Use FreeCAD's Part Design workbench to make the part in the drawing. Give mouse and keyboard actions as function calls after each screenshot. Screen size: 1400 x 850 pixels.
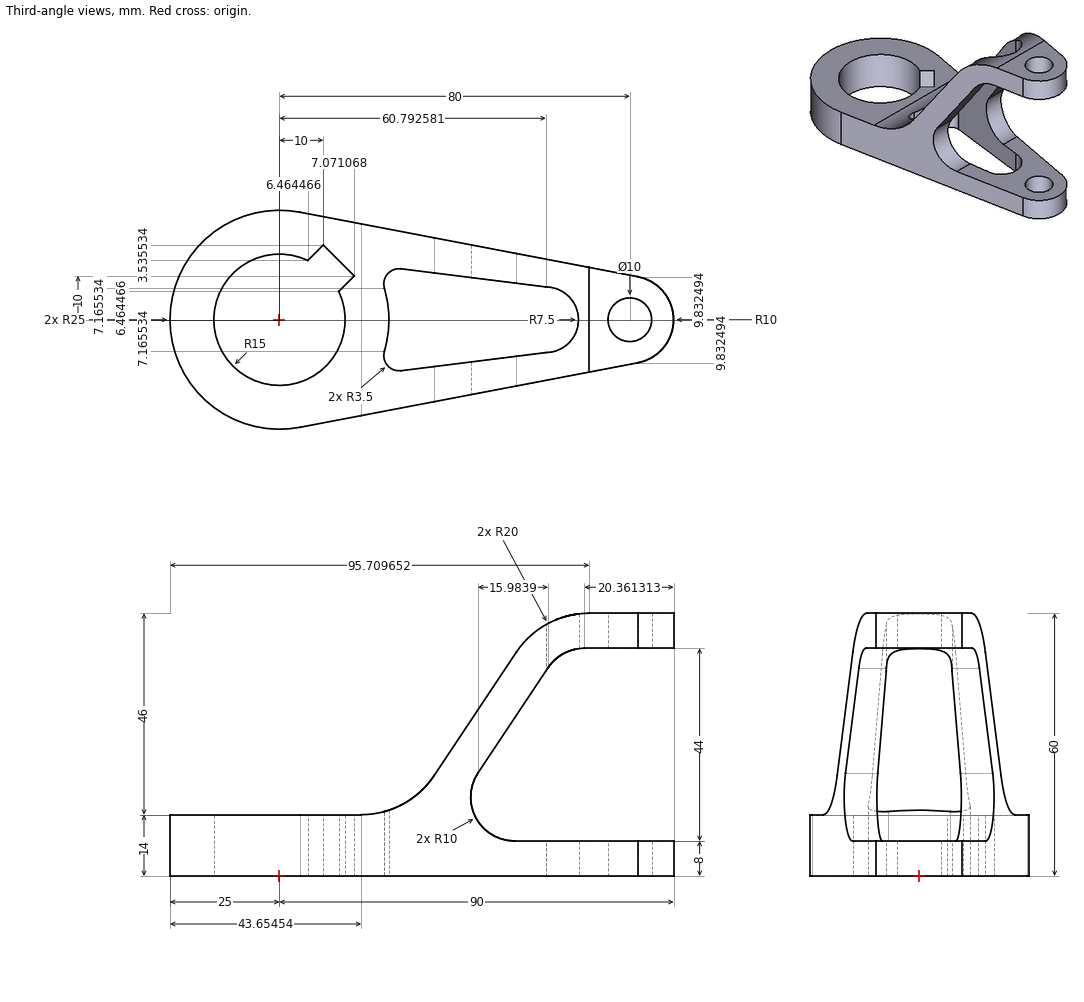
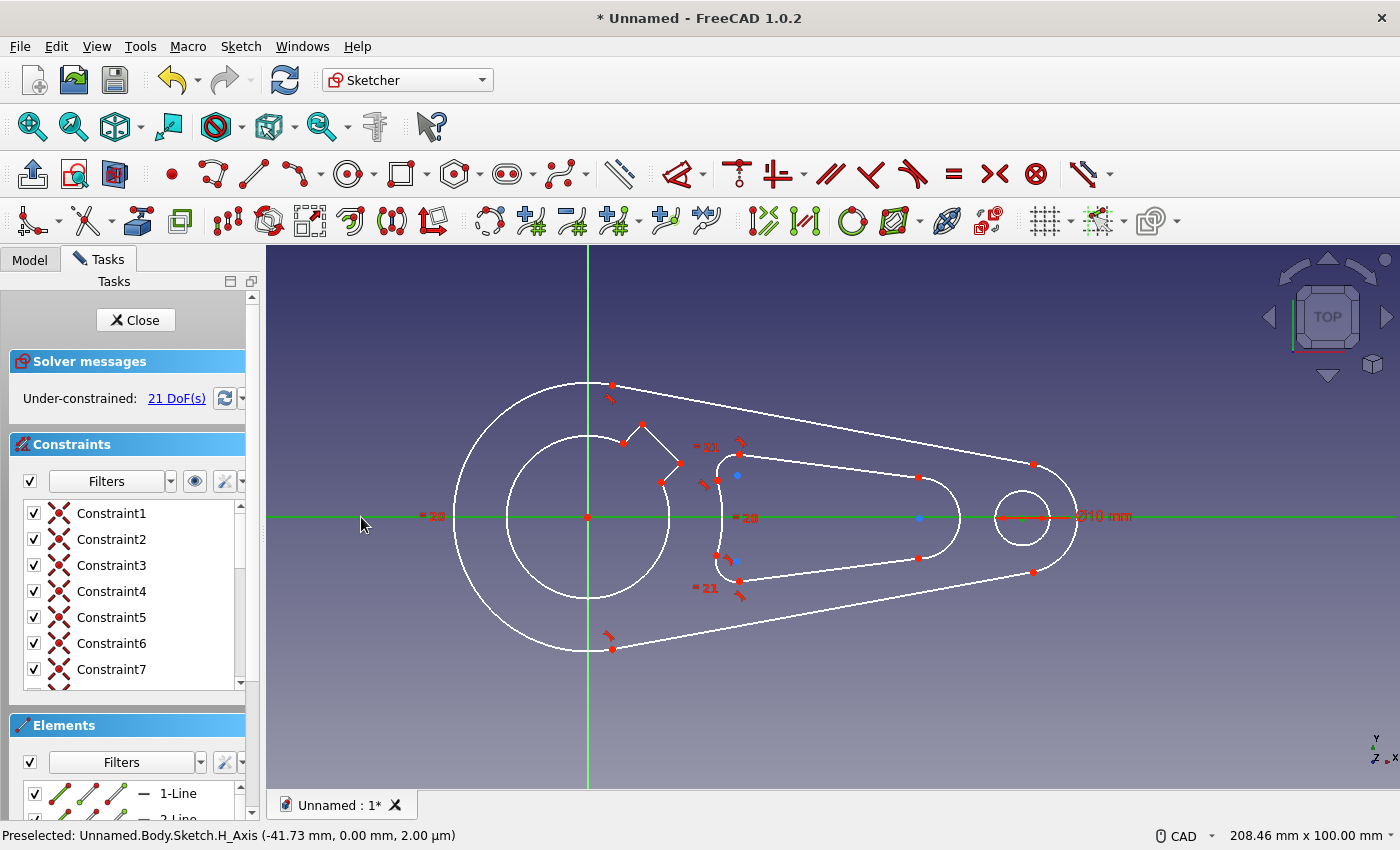
click(737, 174)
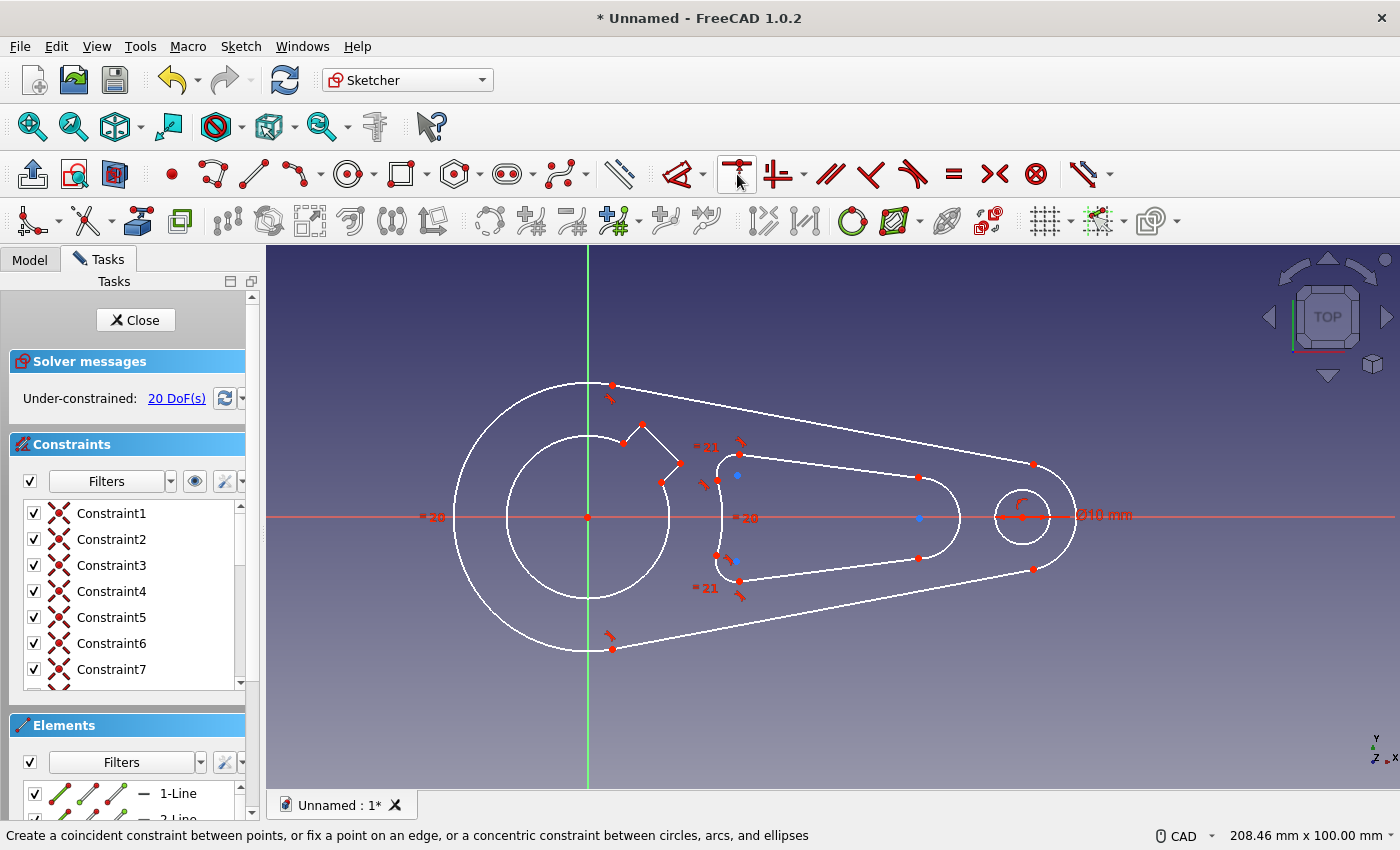
click(920, 518)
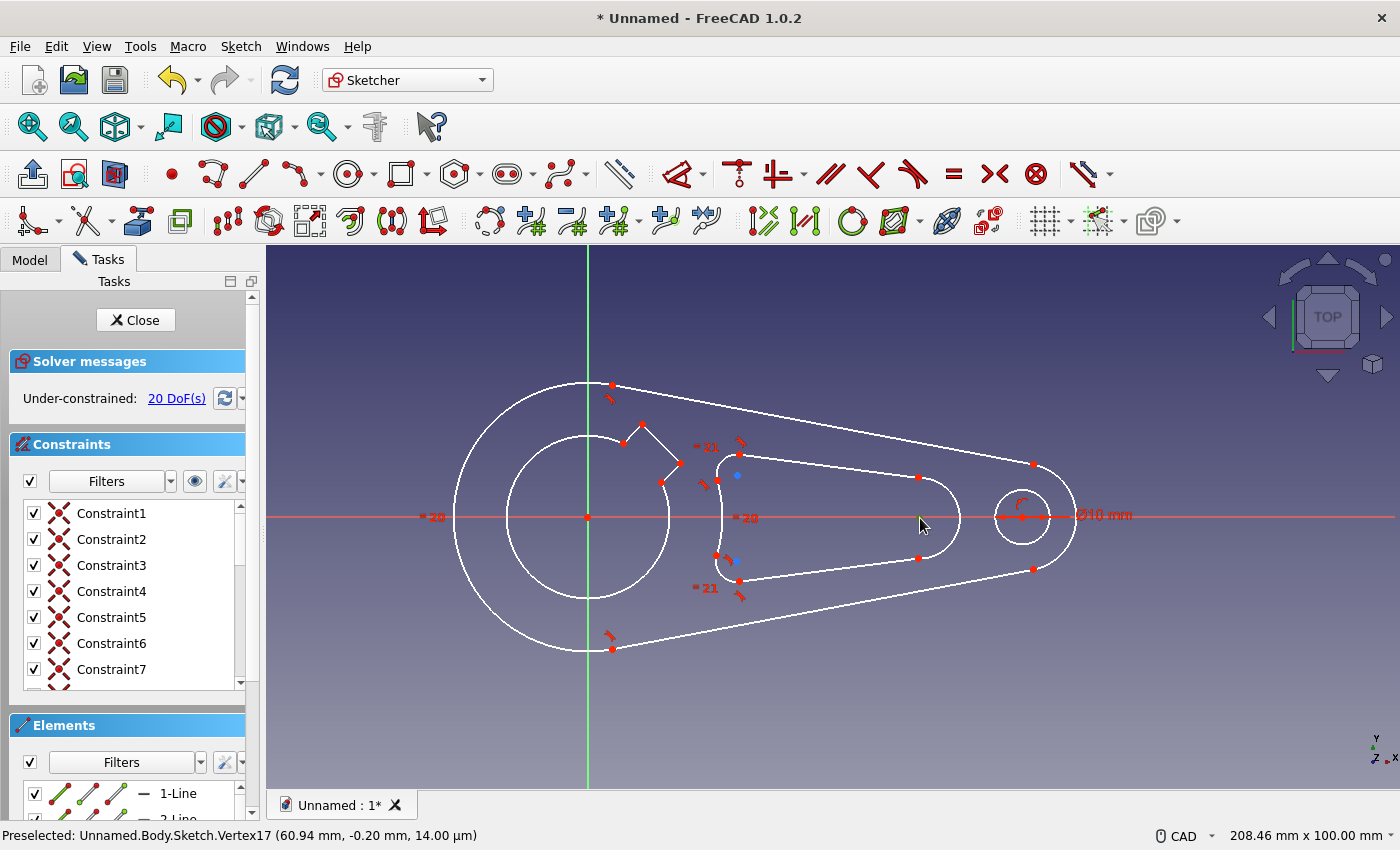
click(361, 517)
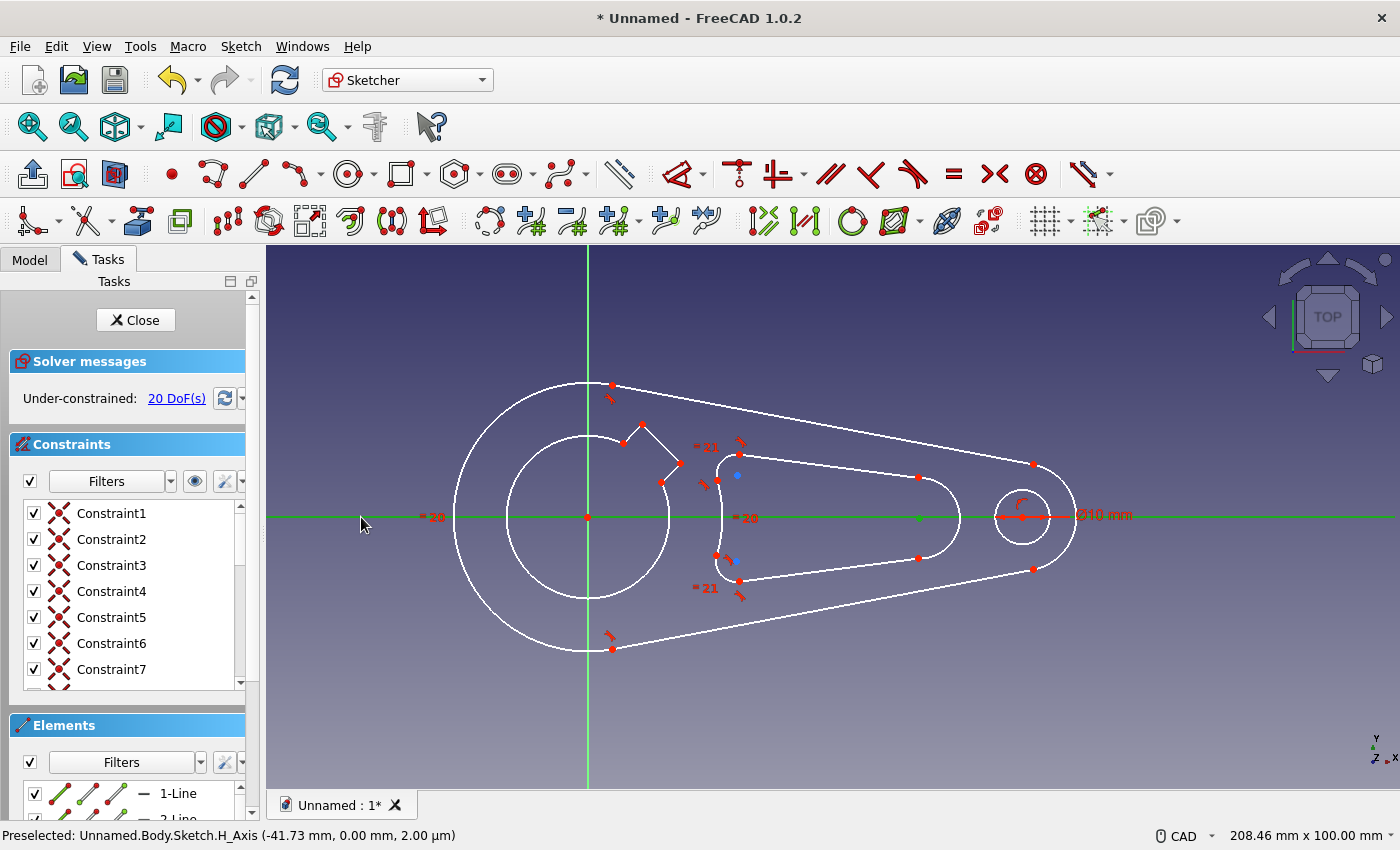
click(737, 174)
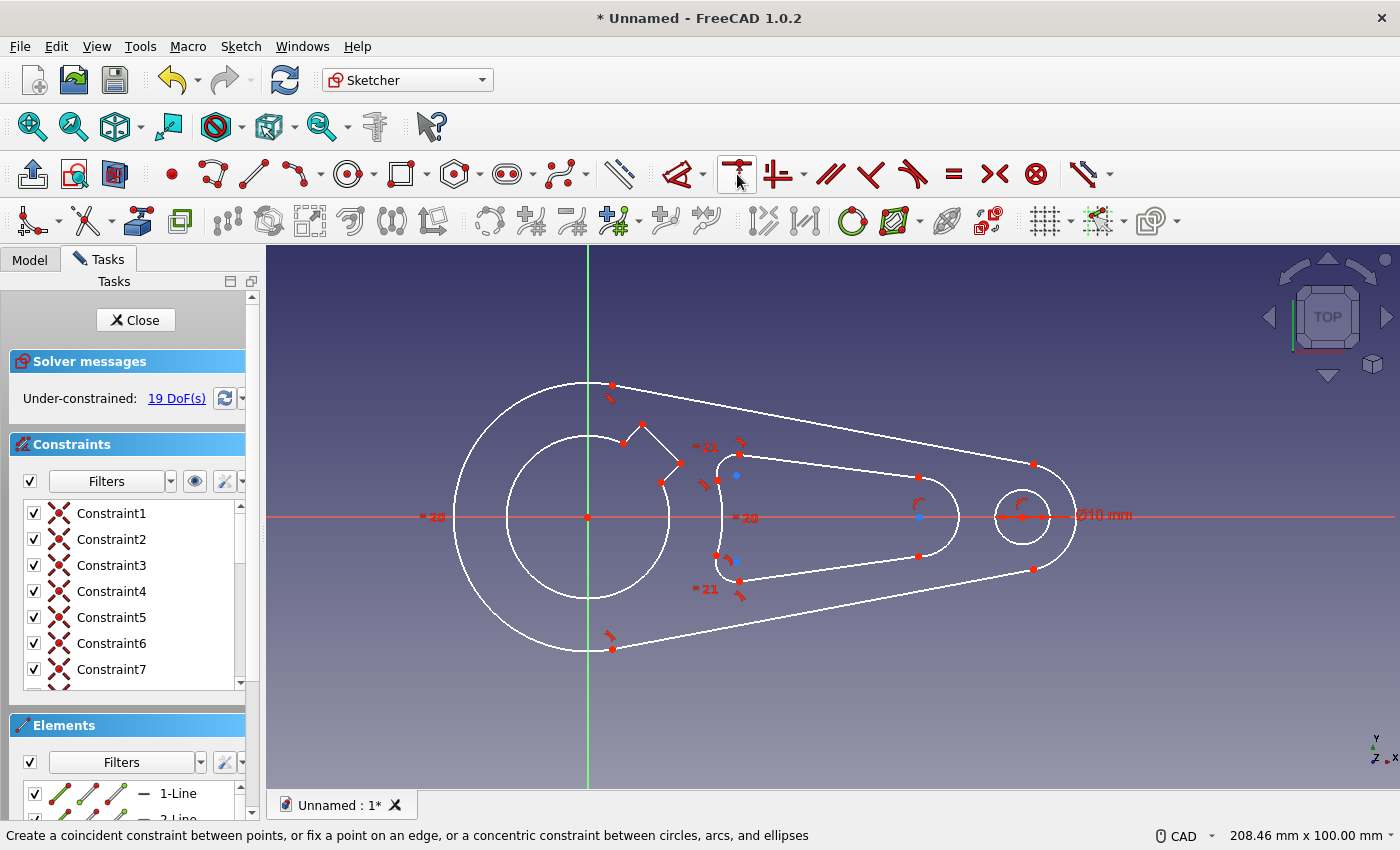
click(485, 430)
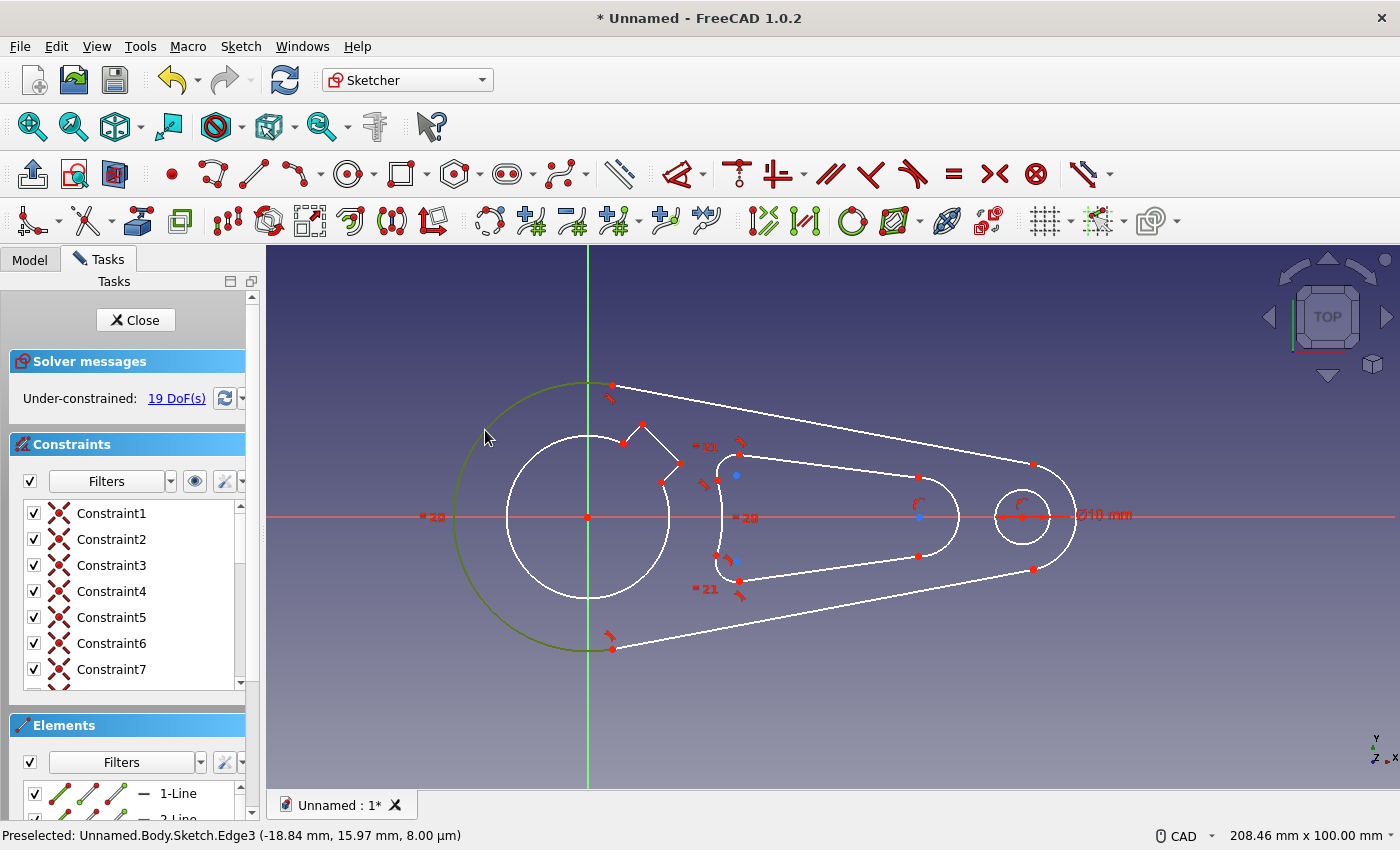
key(k)
key(r)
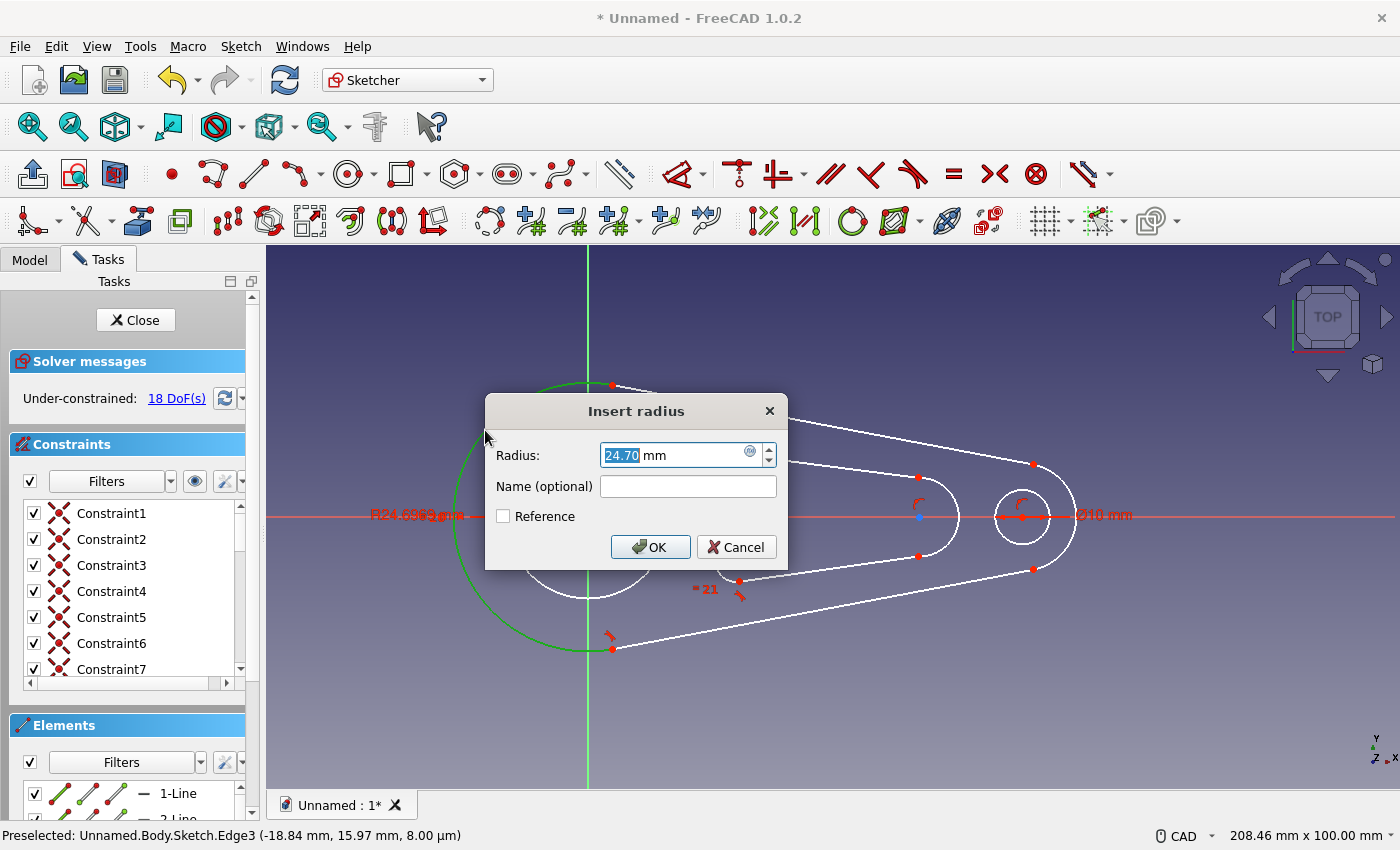
text(25)
key(Return)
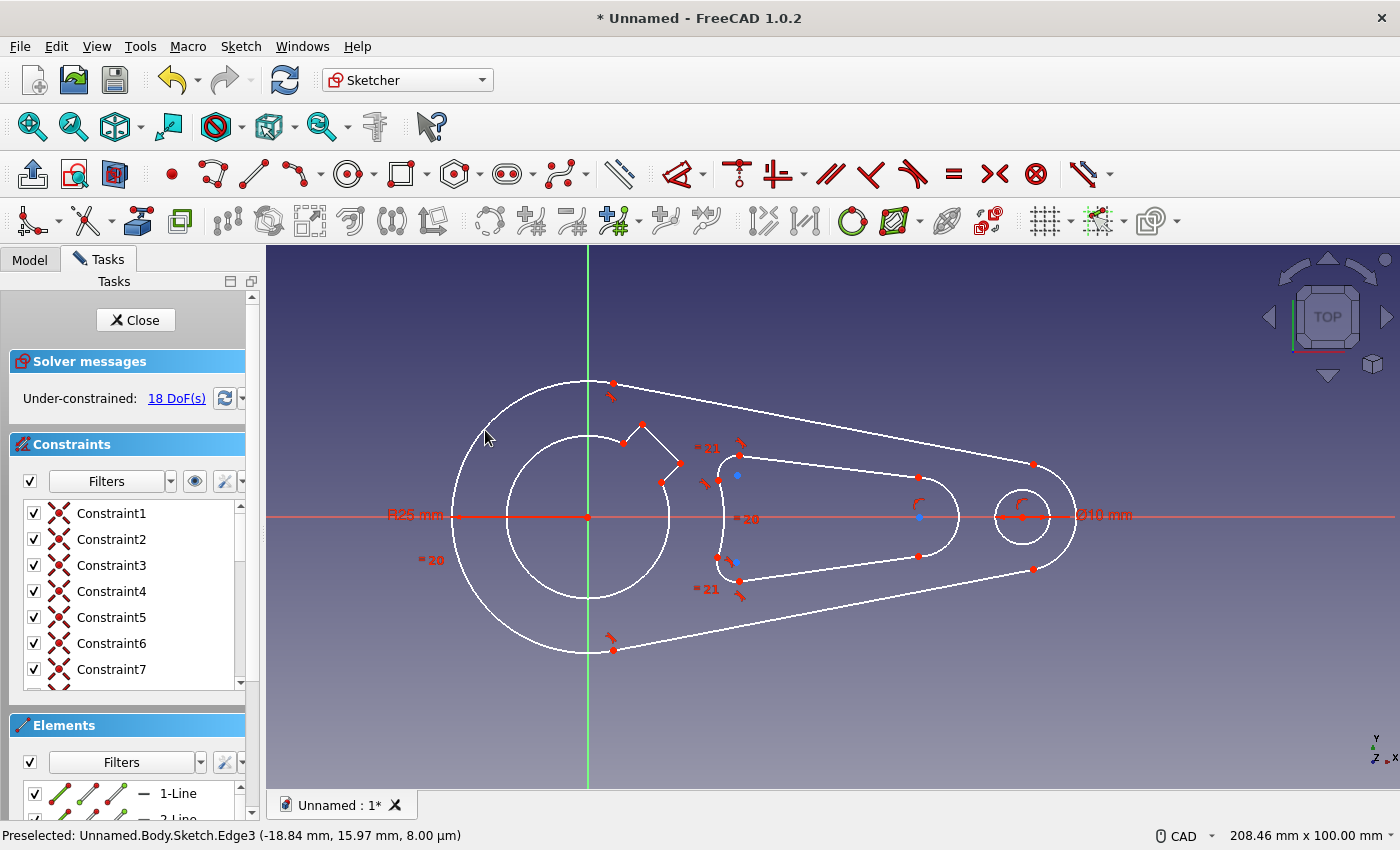
click(1068, 545)